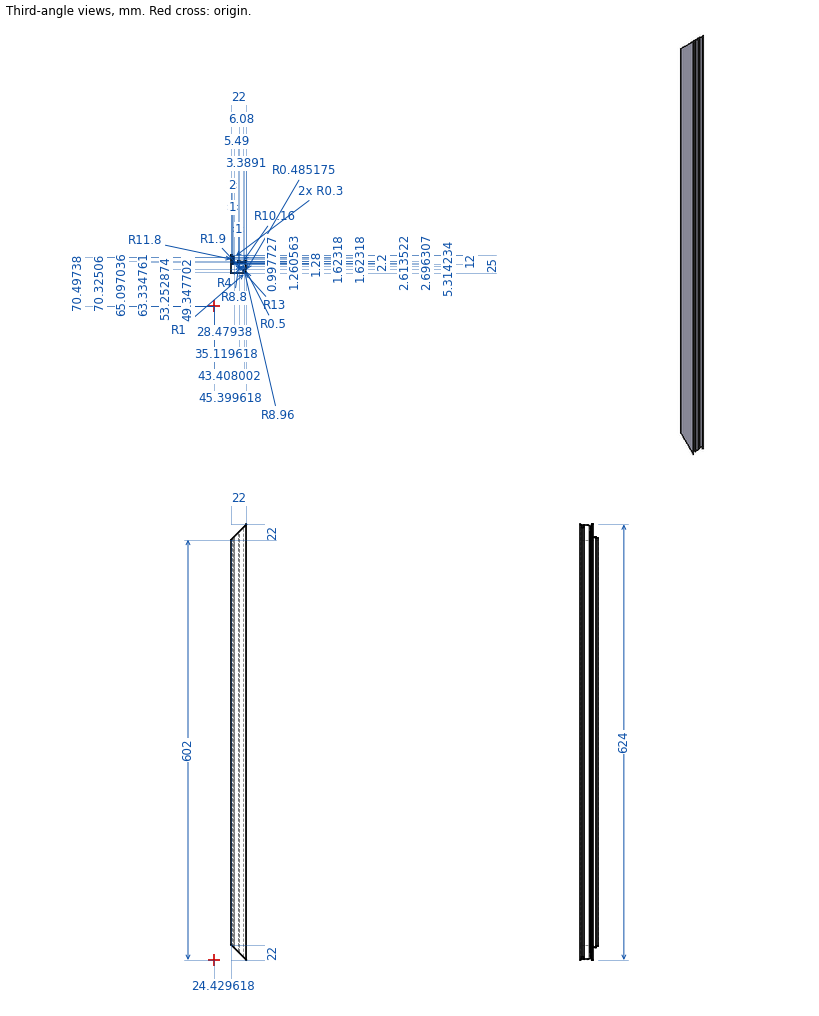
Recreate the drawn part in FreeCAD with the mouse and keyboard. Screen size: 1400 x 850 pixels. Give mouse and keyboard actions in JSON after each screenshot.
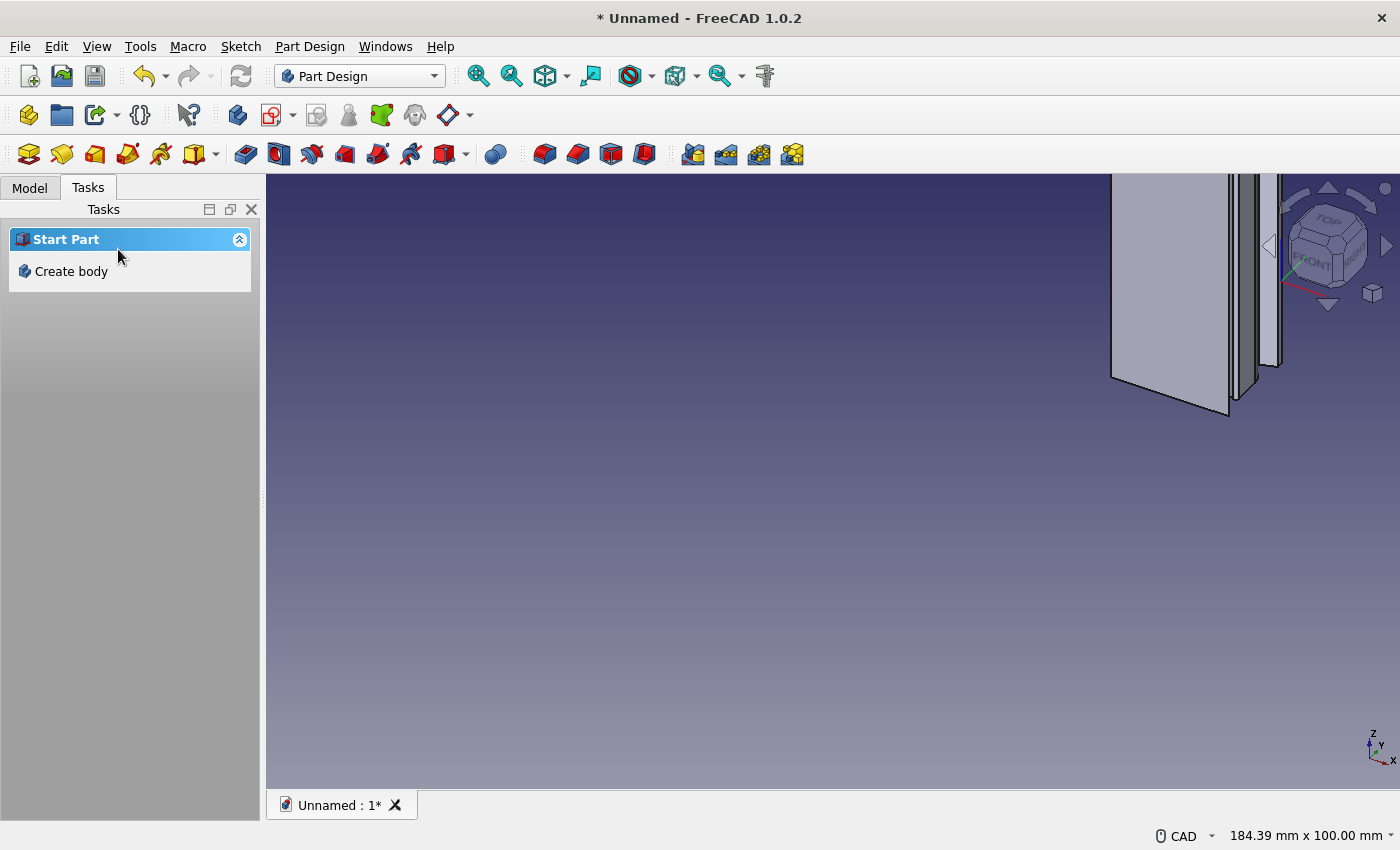
{"action": "key", "text": "v f"}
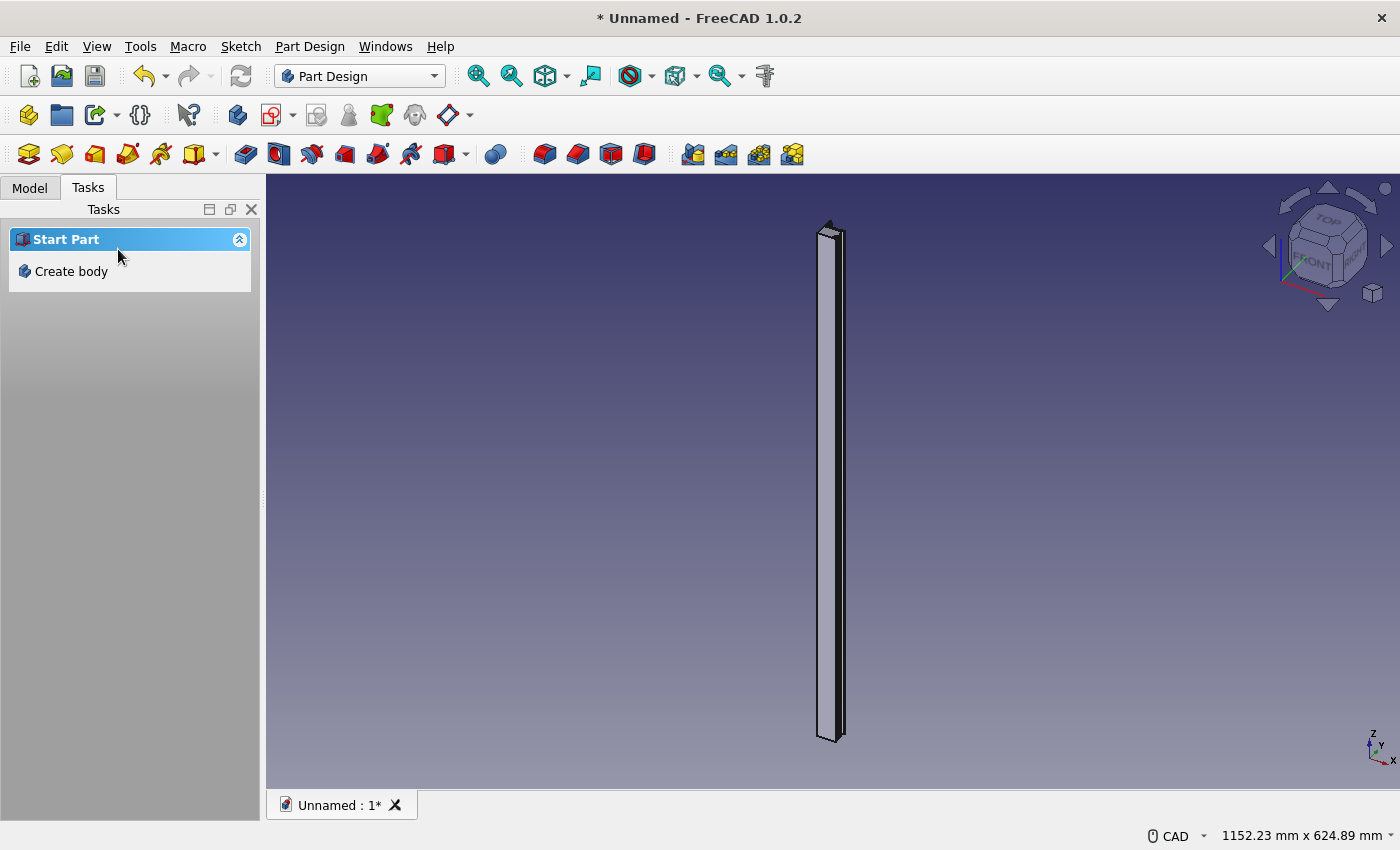
{"action": "left_click", "coordinate": [827, 271]}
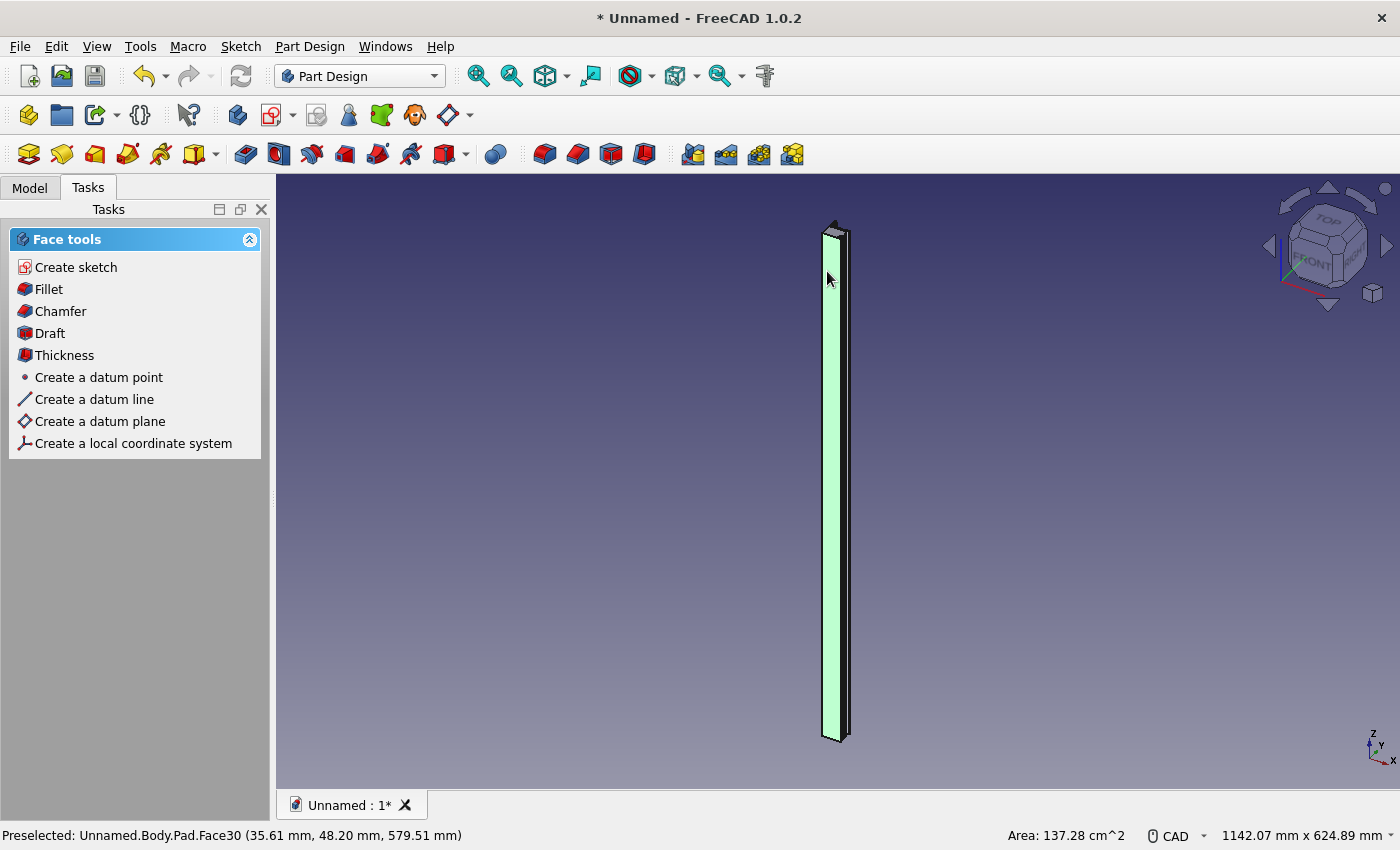
{"action": "left_click", "coordinate": [270, 116]}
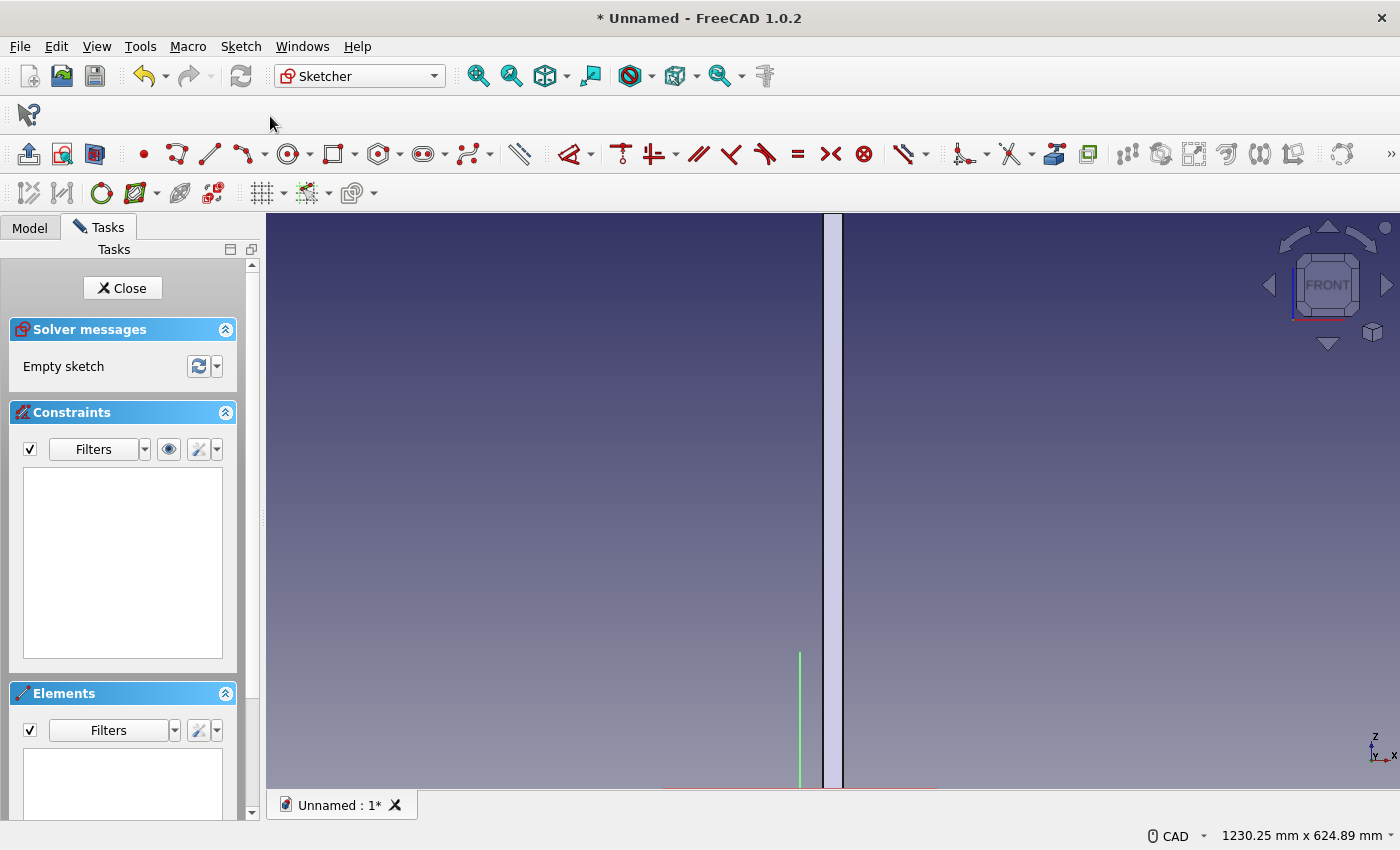
{"action": "scroll", "coordinate": [648, 501], "scroll_direction": "down", "scroll_amount": 2}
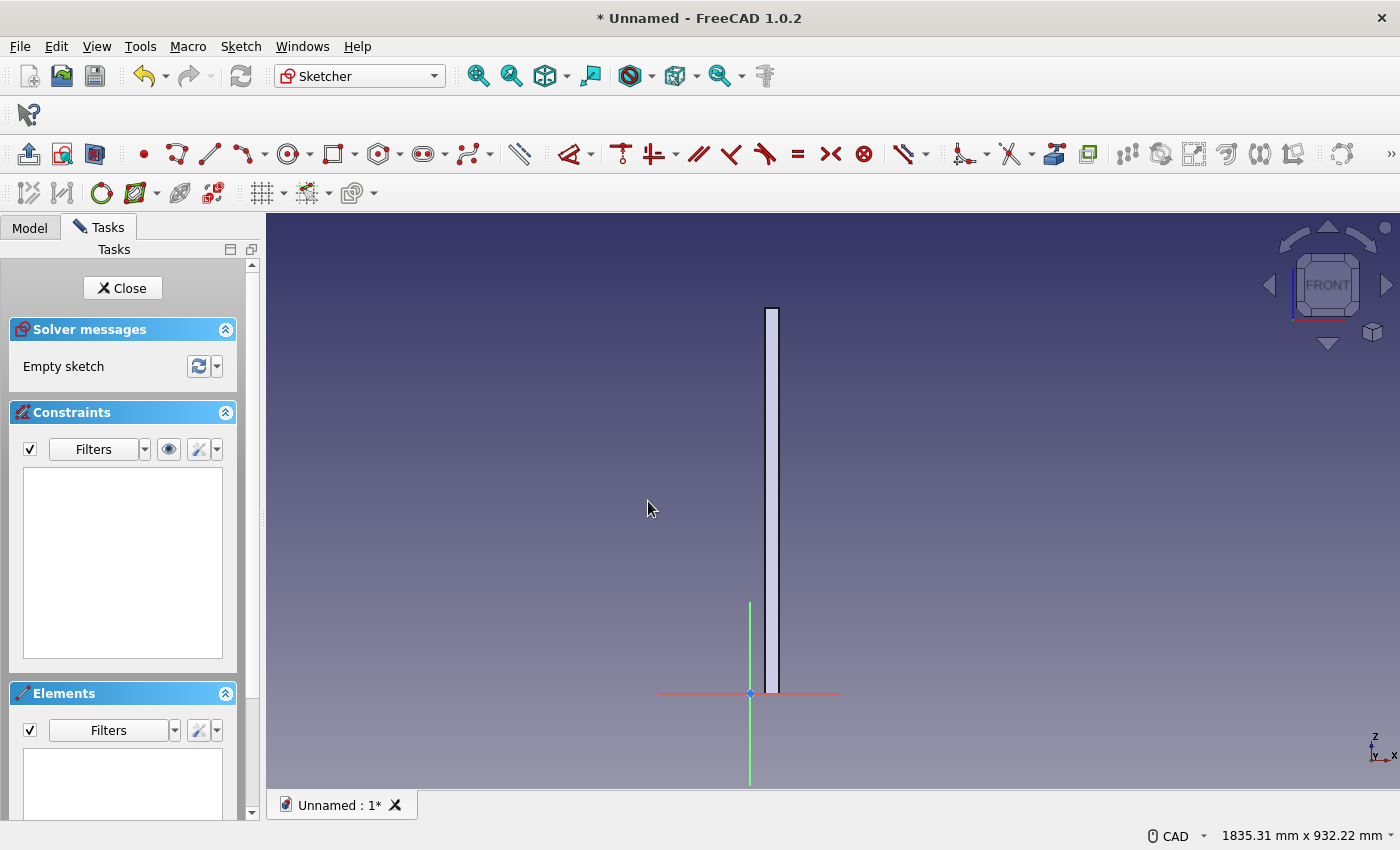
{"action": "left_click", "coordinate": [177, 154]}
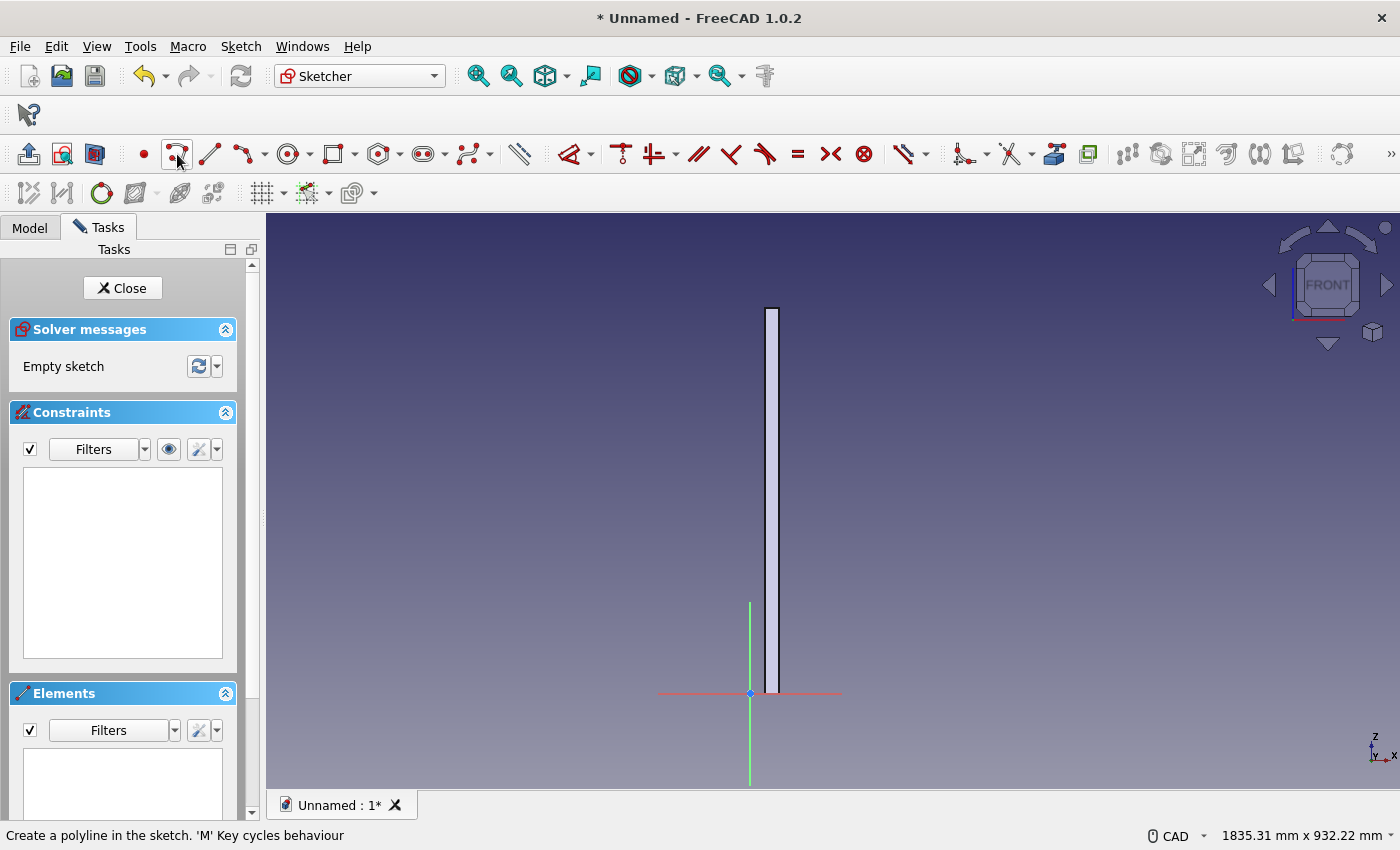
{"action": "left_click", "coordinate": [765, 322]}
{"action": "left_click", "coordinate": [779, 308]}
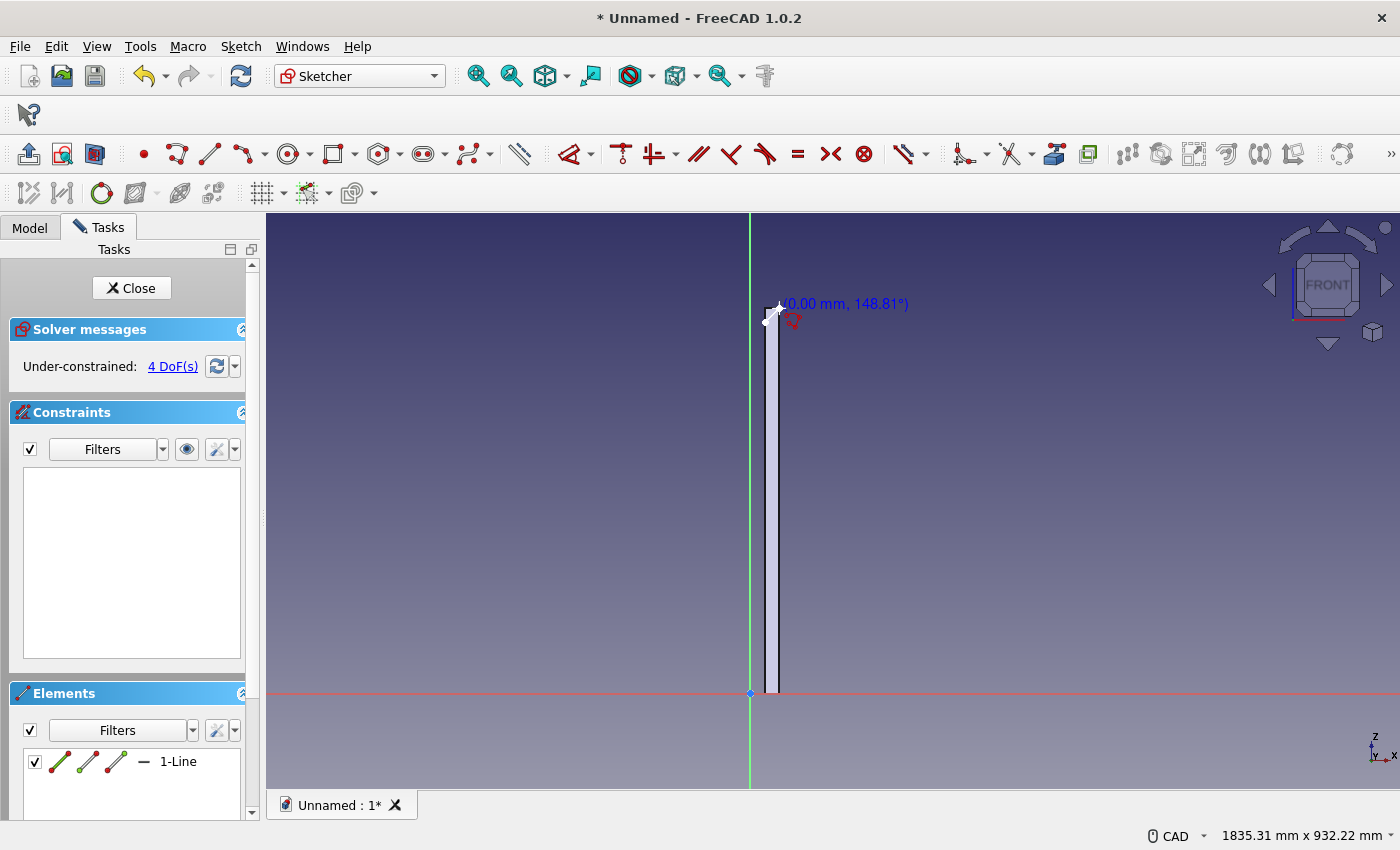
{"action": "scroll", "coordinate": [765, 308], "scroll_direction": "up", "scroll_amount": 3}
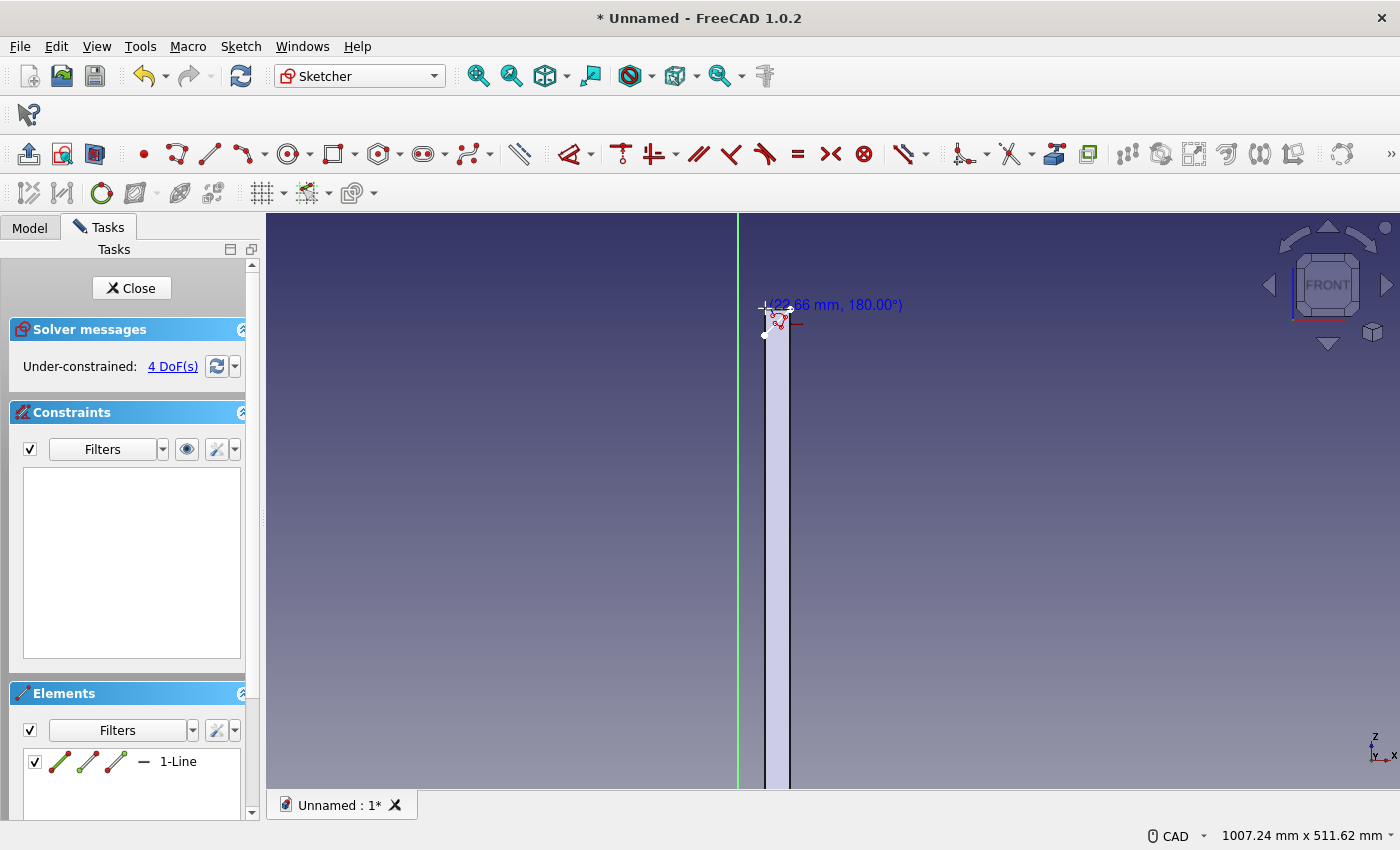
{"action": "left_click", "coordinate": [765, 308]}
{"action": "left_click", "coordinate": [765, 335]}